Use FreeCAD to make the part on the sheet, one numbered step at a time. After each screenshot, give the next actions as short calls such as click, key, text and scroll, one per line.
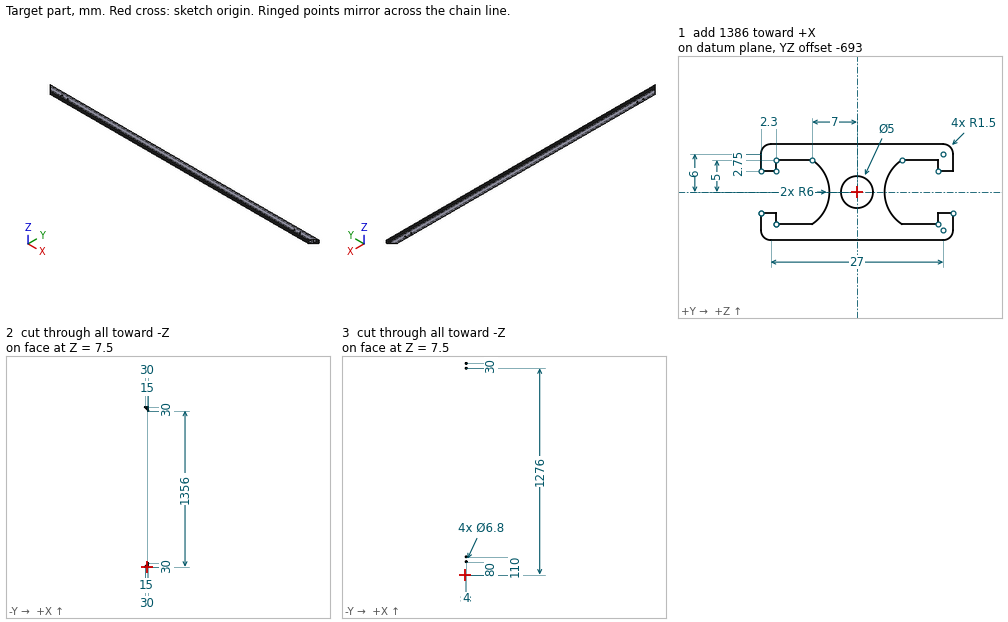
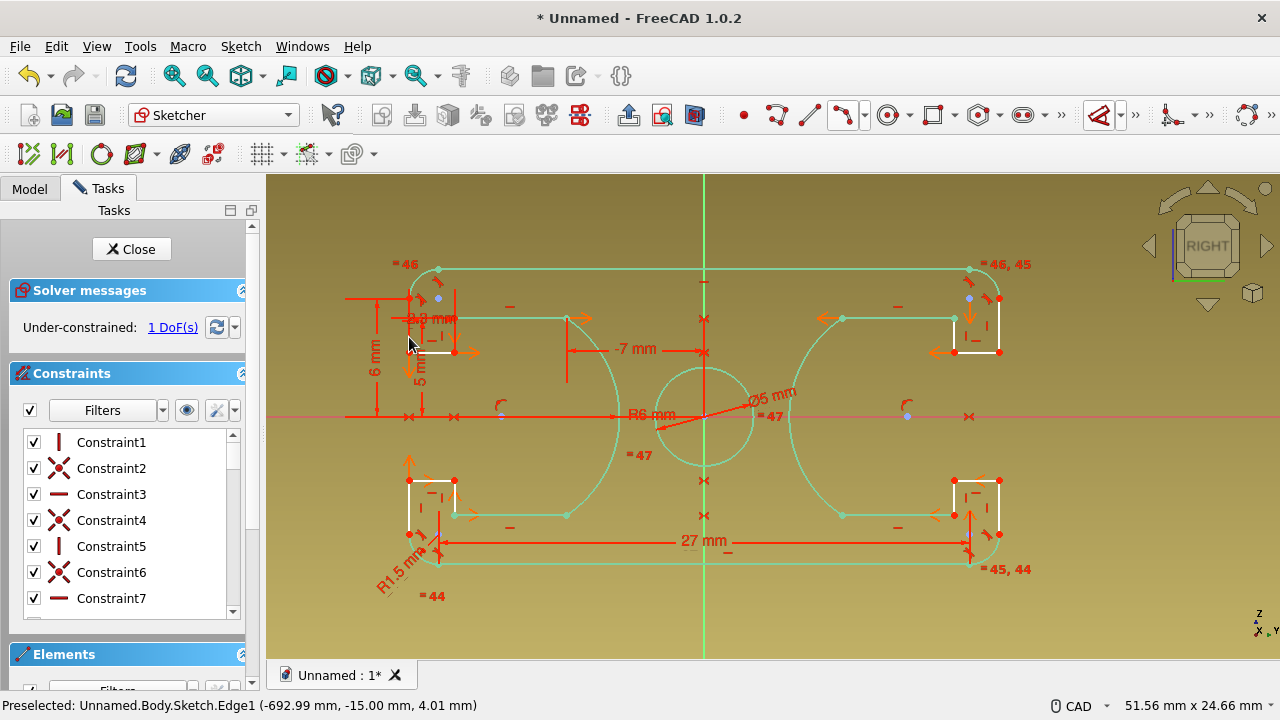
key(i)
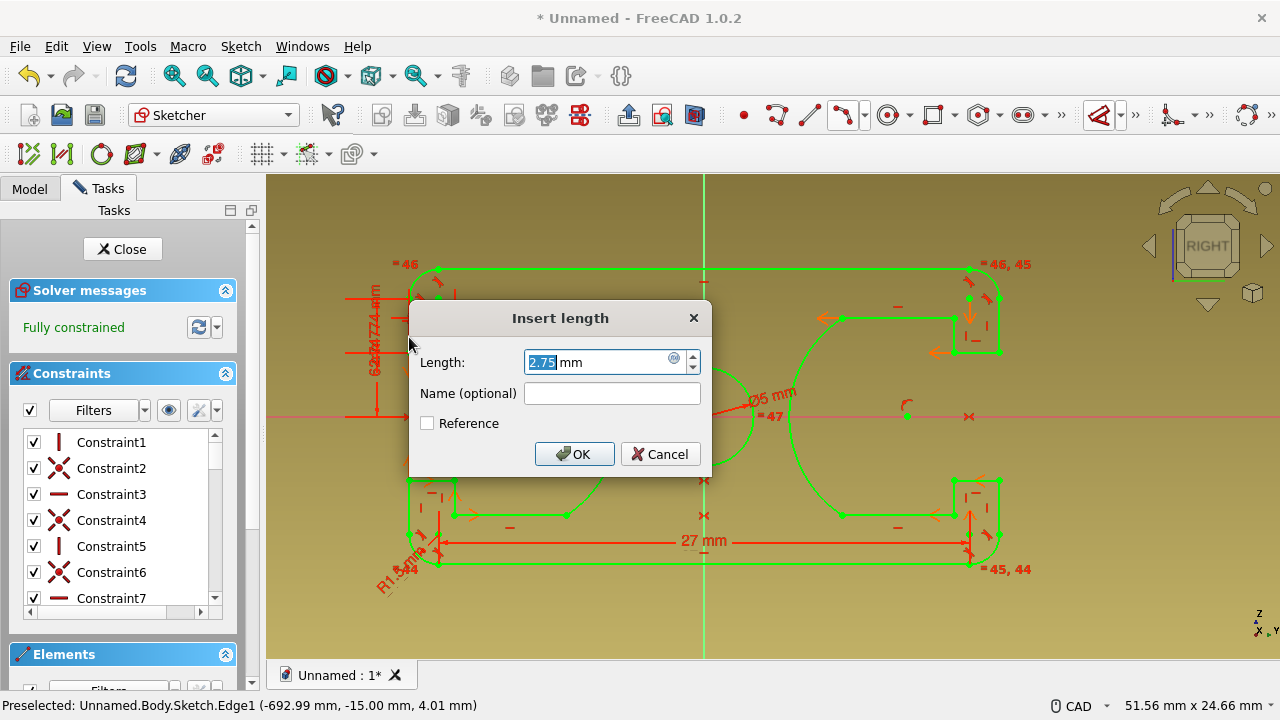
text(2.75)
key(Return)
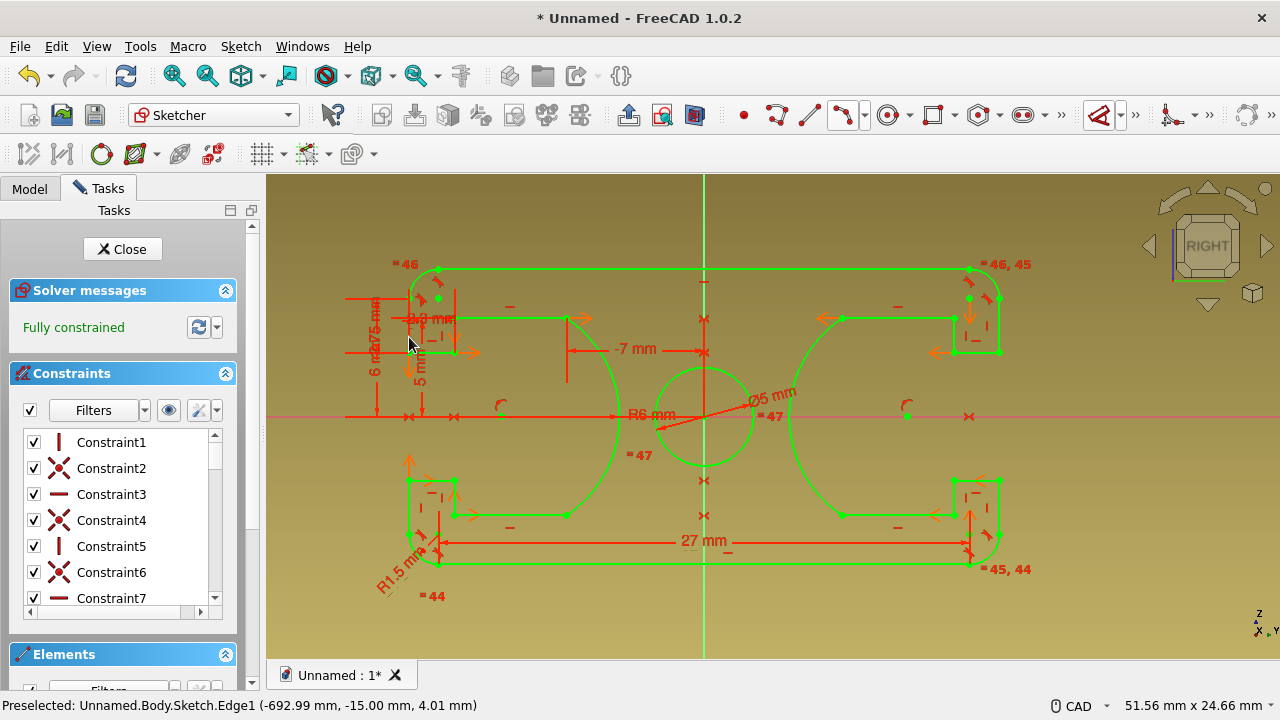
click(123, 249)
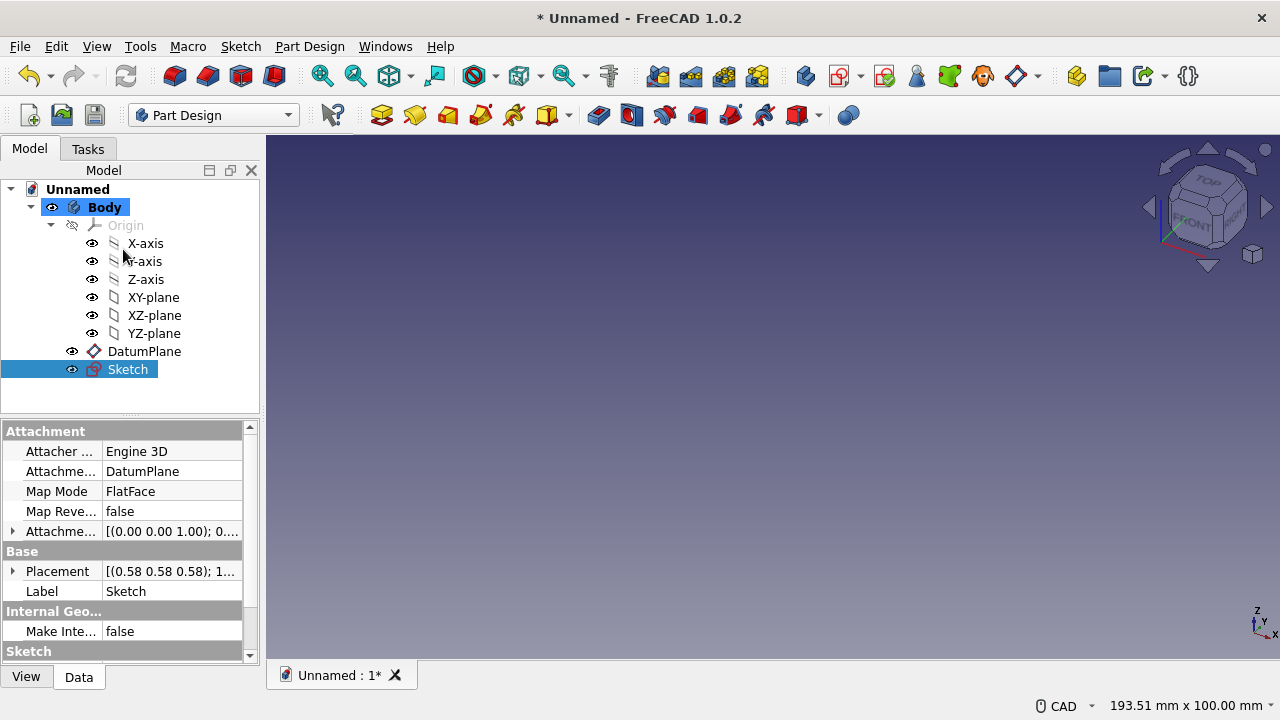
click(382, 116)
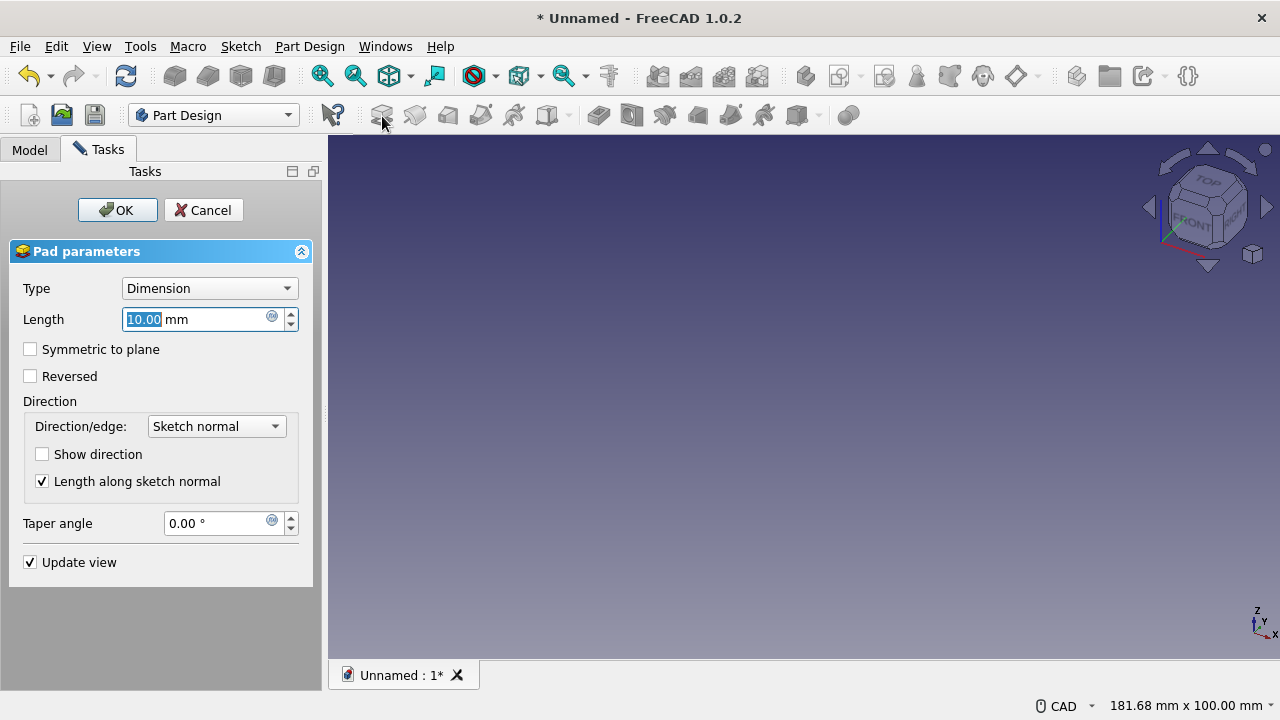
text(1386)
key(Tab)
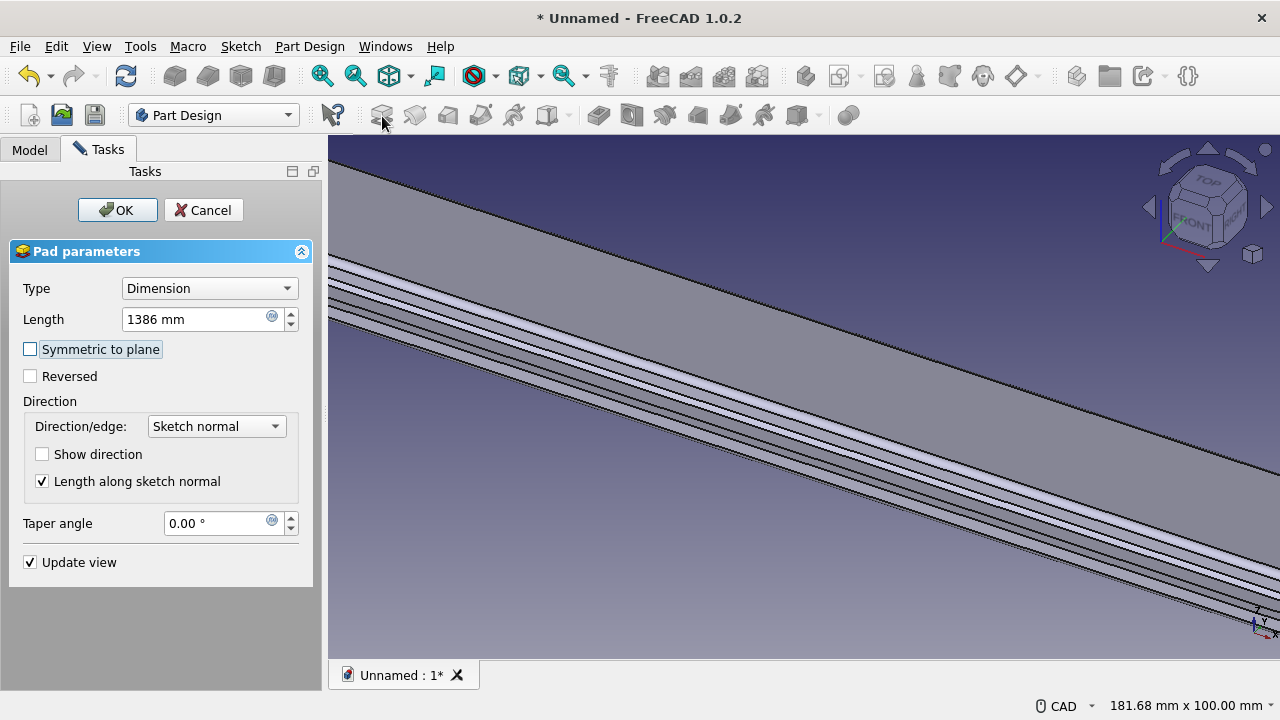
click(118, 210)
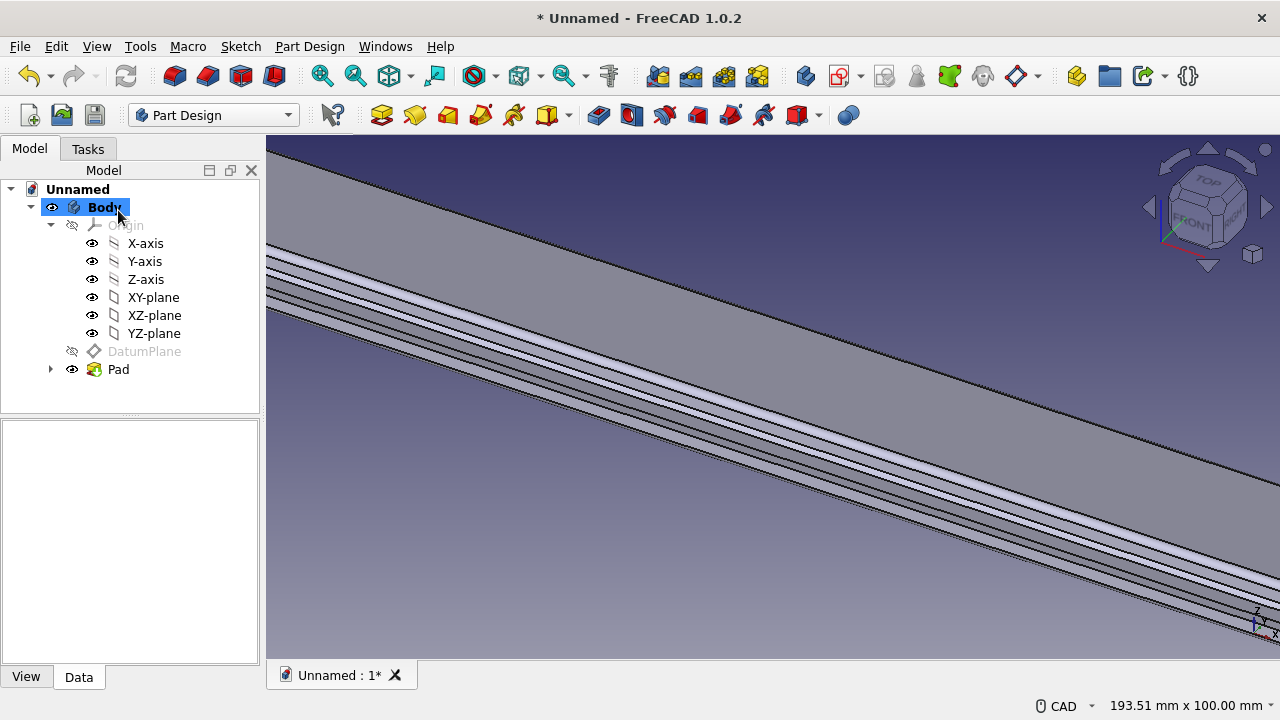
key(v)
key(f)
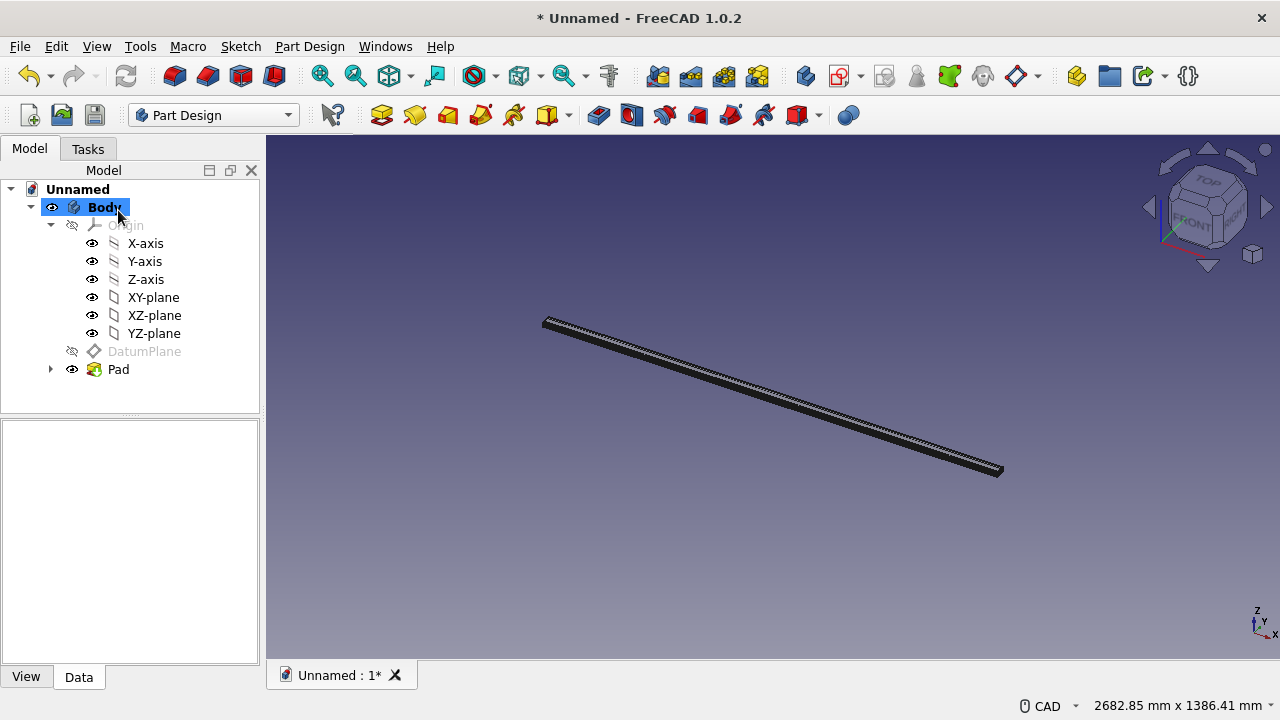
scroll(773, 394, up, 5)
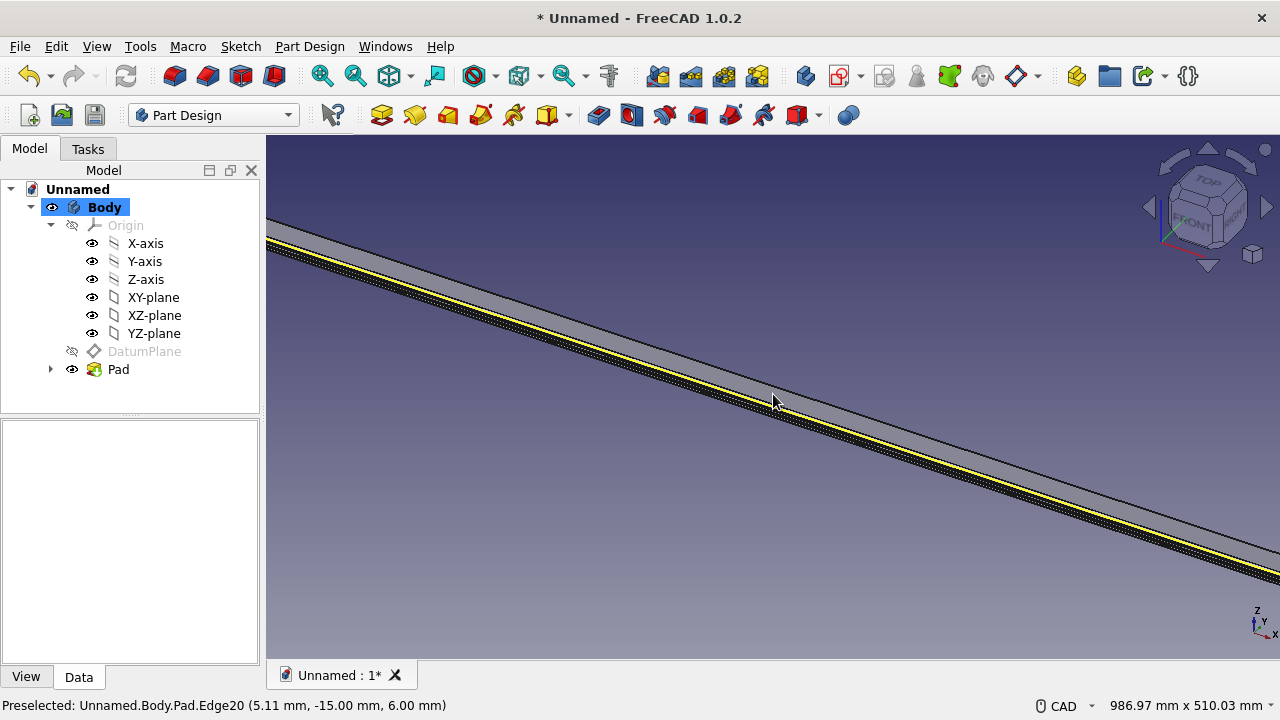
click(323, 76)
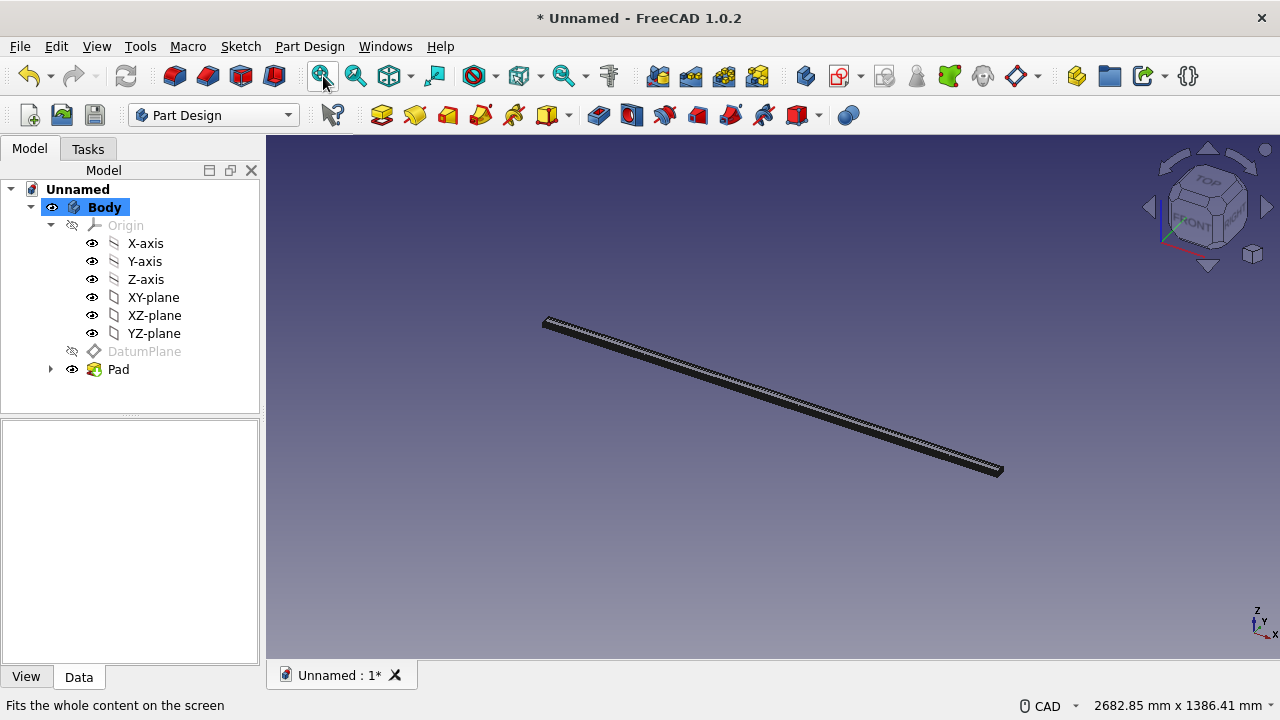
key(0)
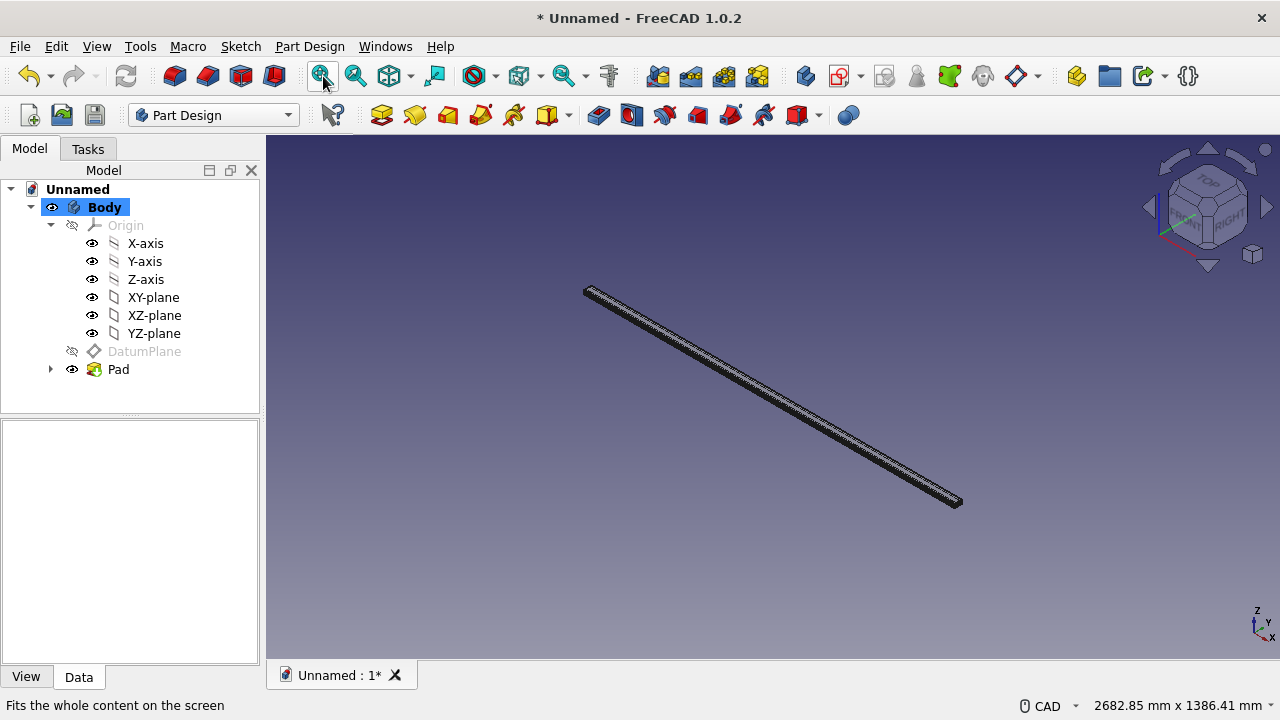
click(323, 76)